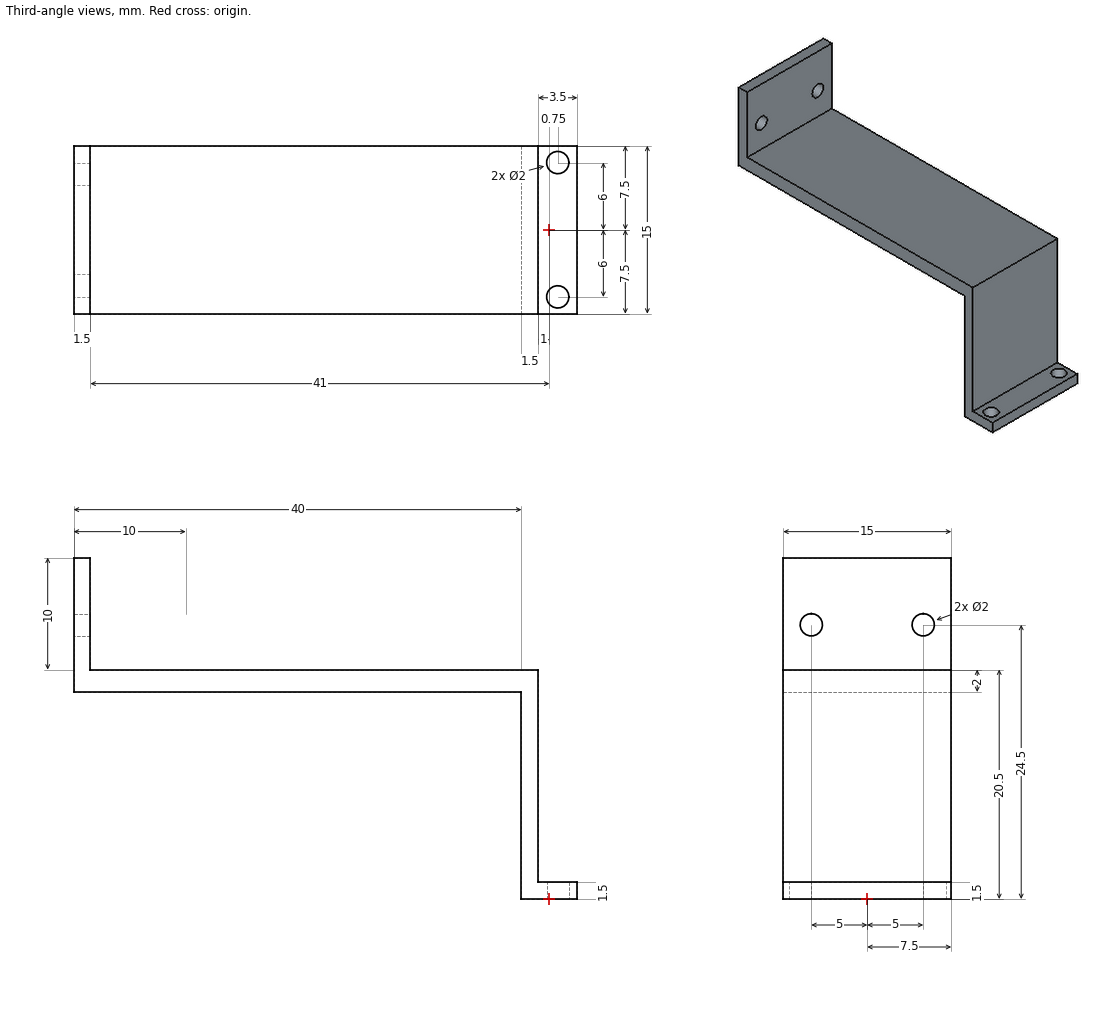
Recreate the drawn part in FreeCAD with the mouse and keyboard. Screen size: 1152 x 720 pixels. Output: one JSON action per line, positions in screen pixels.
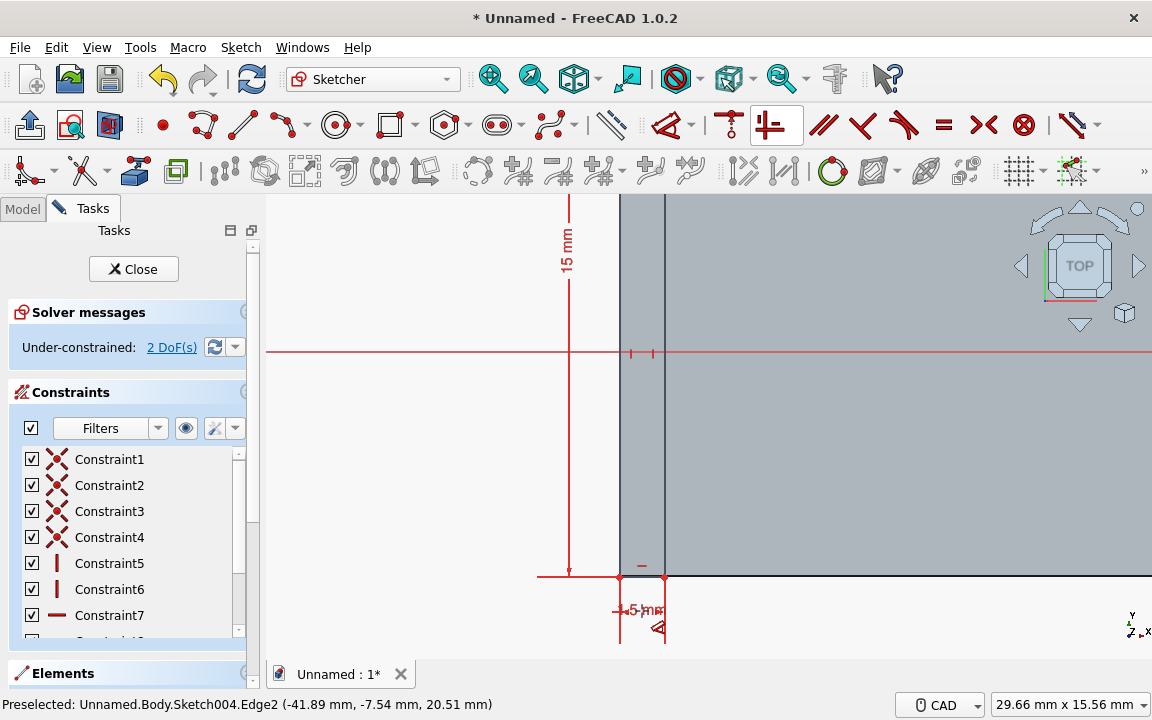
{"action": "left_click", "coordinate": [665, 577]}
{"action": "left_click", "coordinate": [826, 611]}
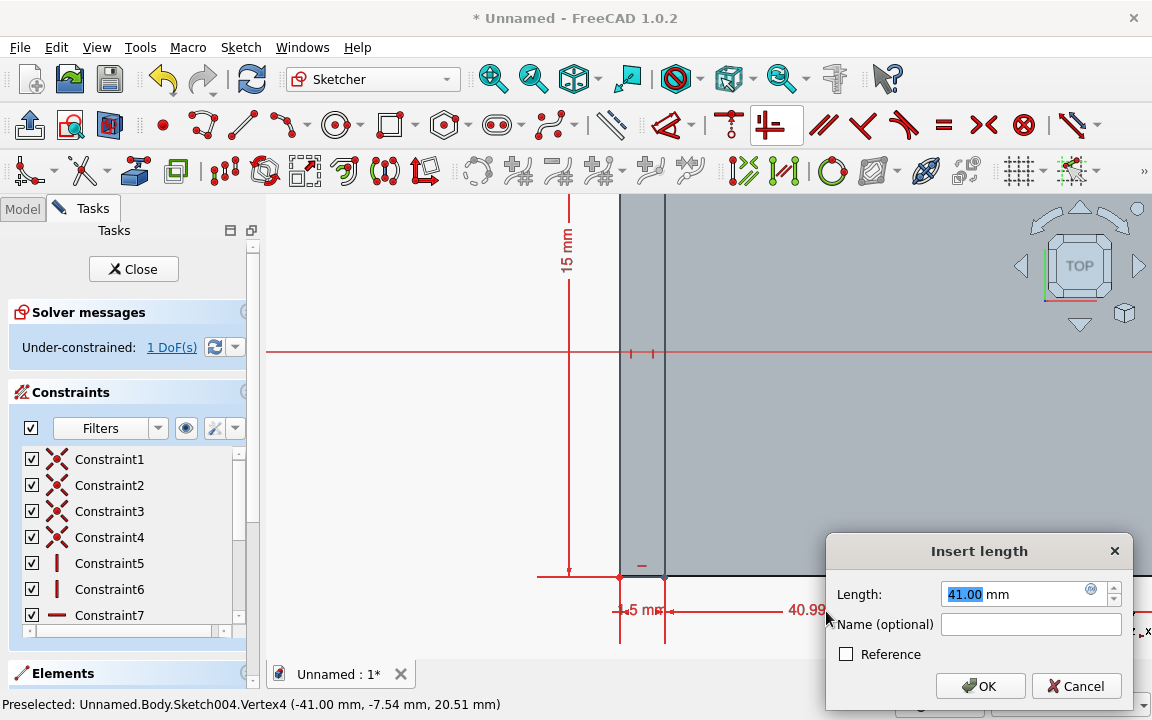
{"action": "type", "text": "41"}
{"action": "key", "text": "Return"}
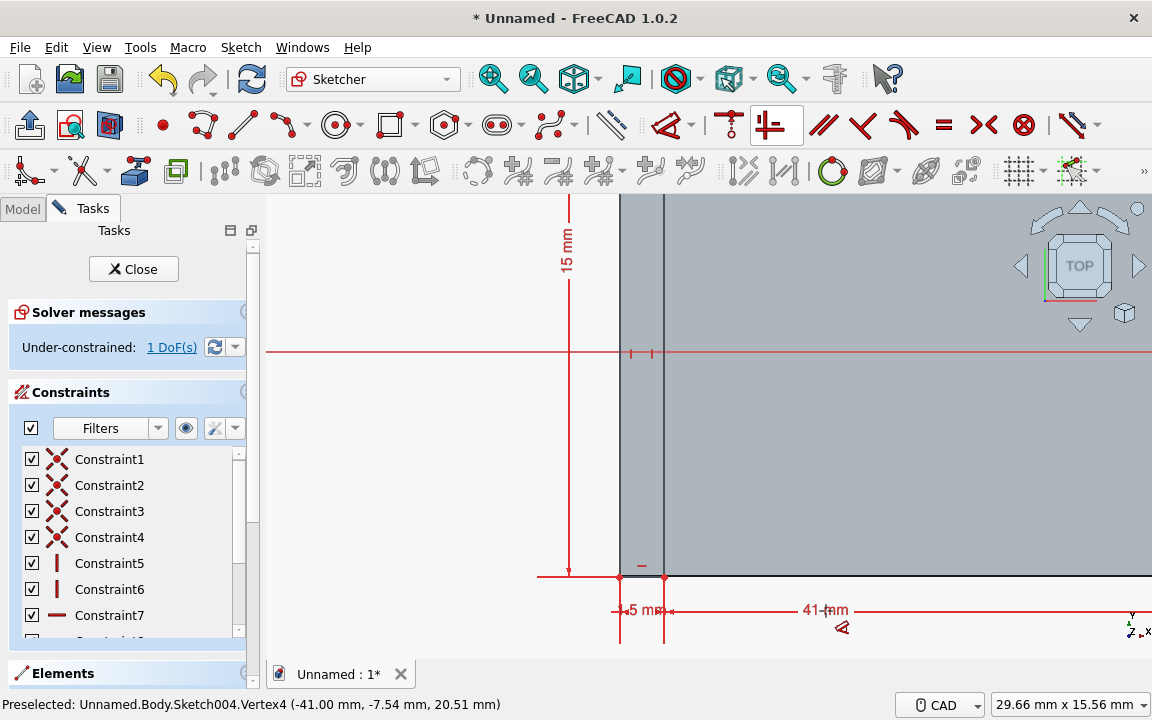
{"action": "scroll", "coordinate": [637, 578], "scroll_direction": "down", "scroll_amount": 2}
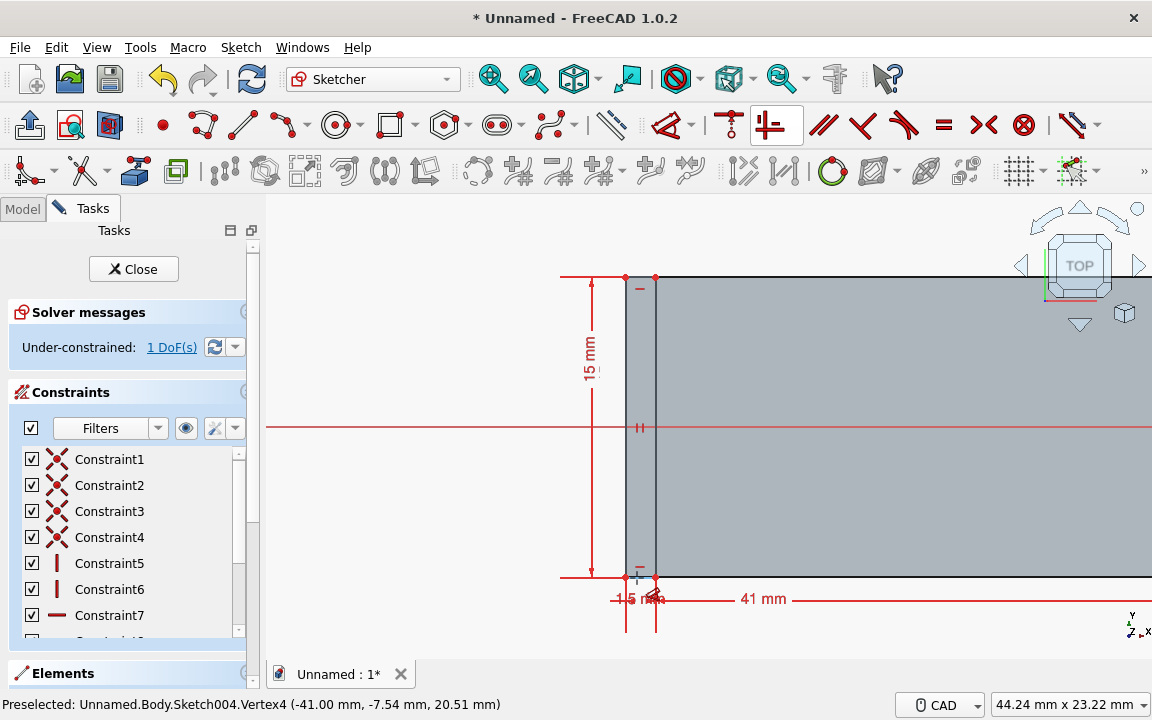
{"action": "left_click", "coordinate": [626, 277]}
{"action": "left_click", "coordinate": [592, 318]}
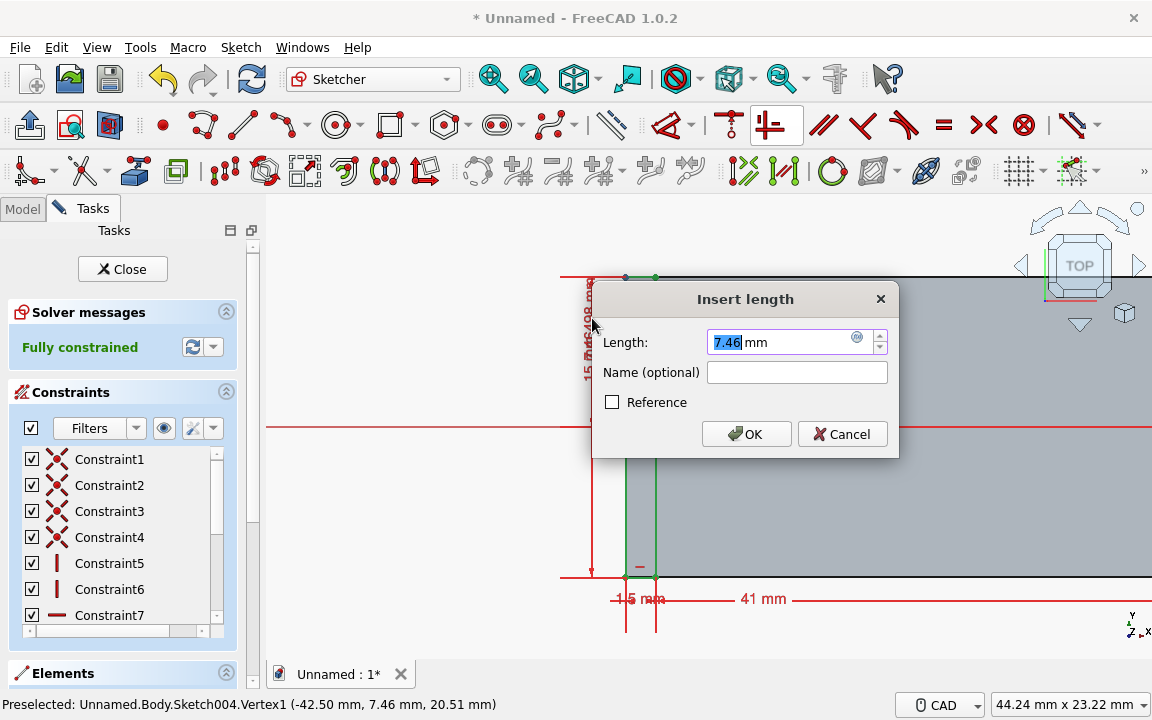
{"action": "type", "text": "7.5"}
{"action": "key", "text": "Return"}
{"action": "key", "text": "Escape"}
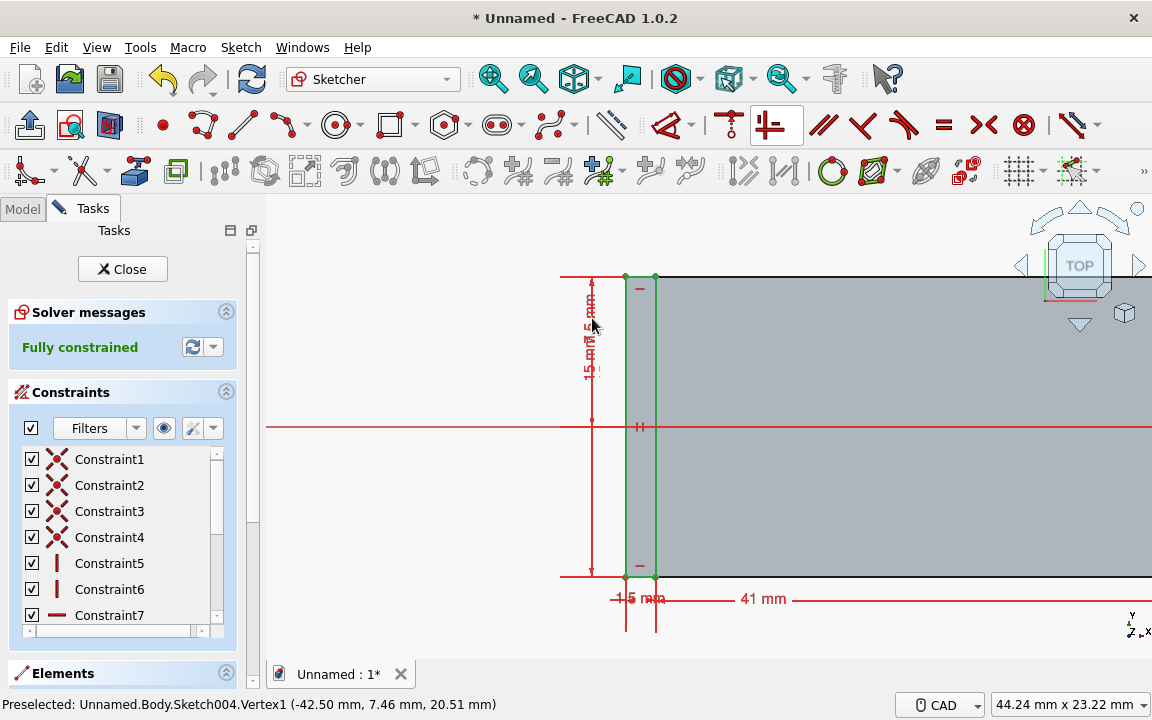
{"action": "left_click", "coordinate": [123, 269]}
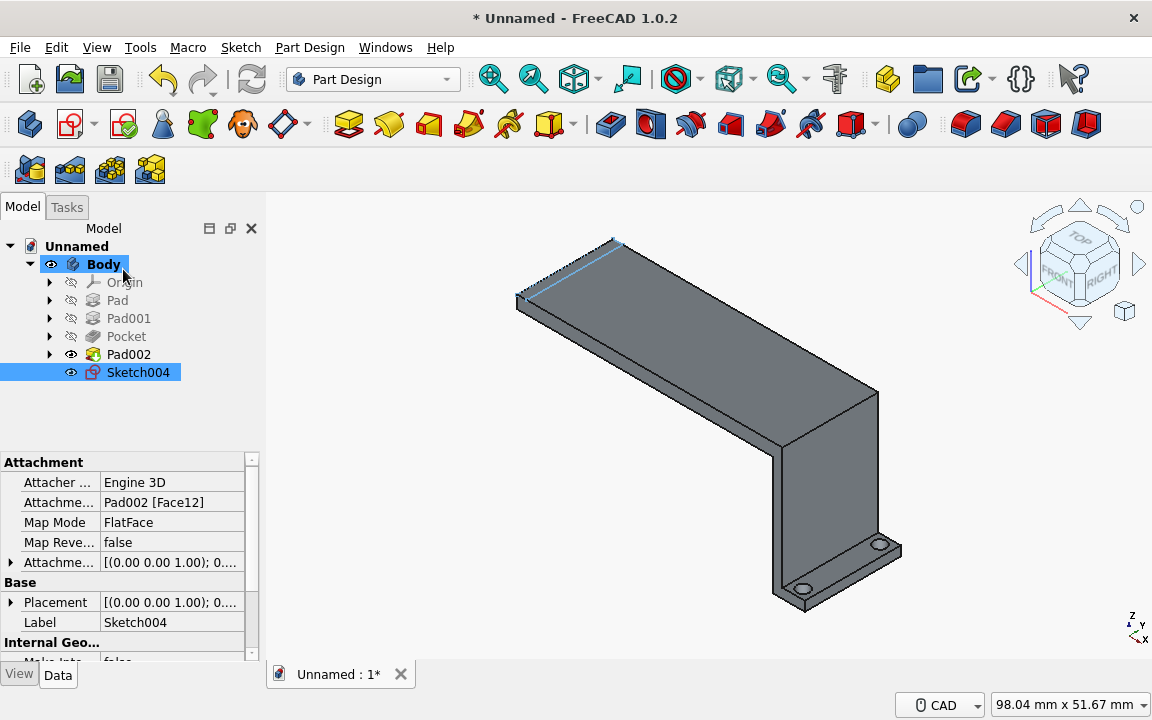
{"action": "left_click", "coordinate": [350, 124]}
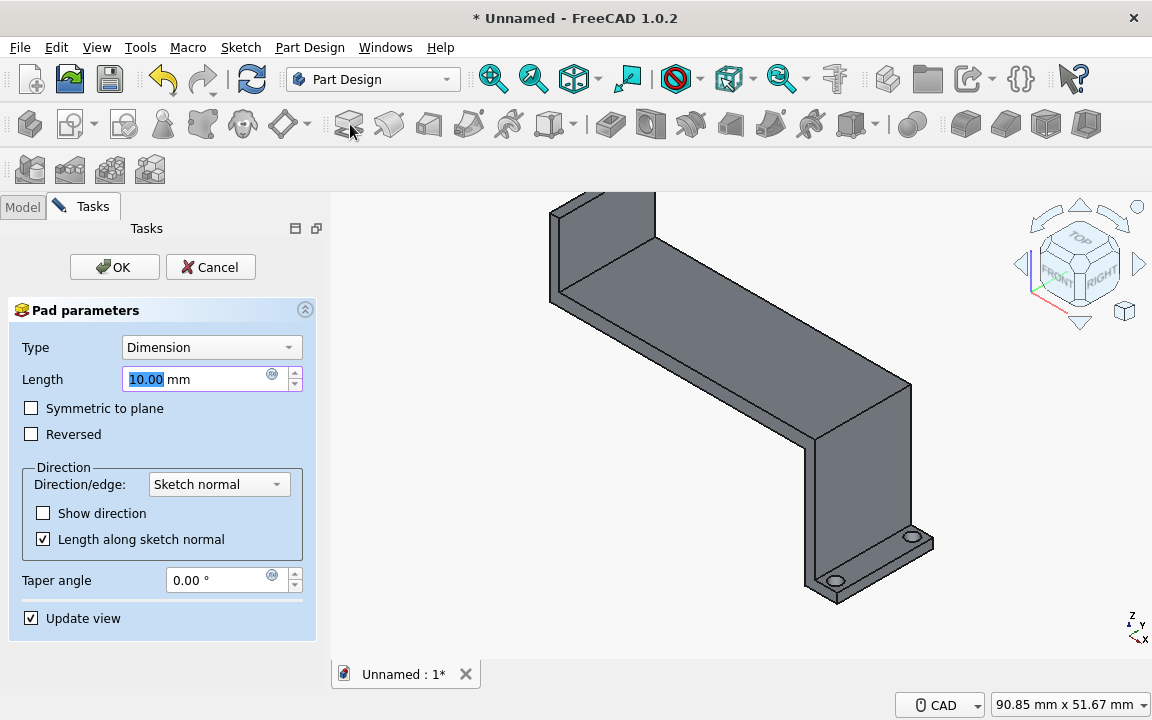
{"action": "type", "text": "10"}
{"action": "key", "text": "Tab"}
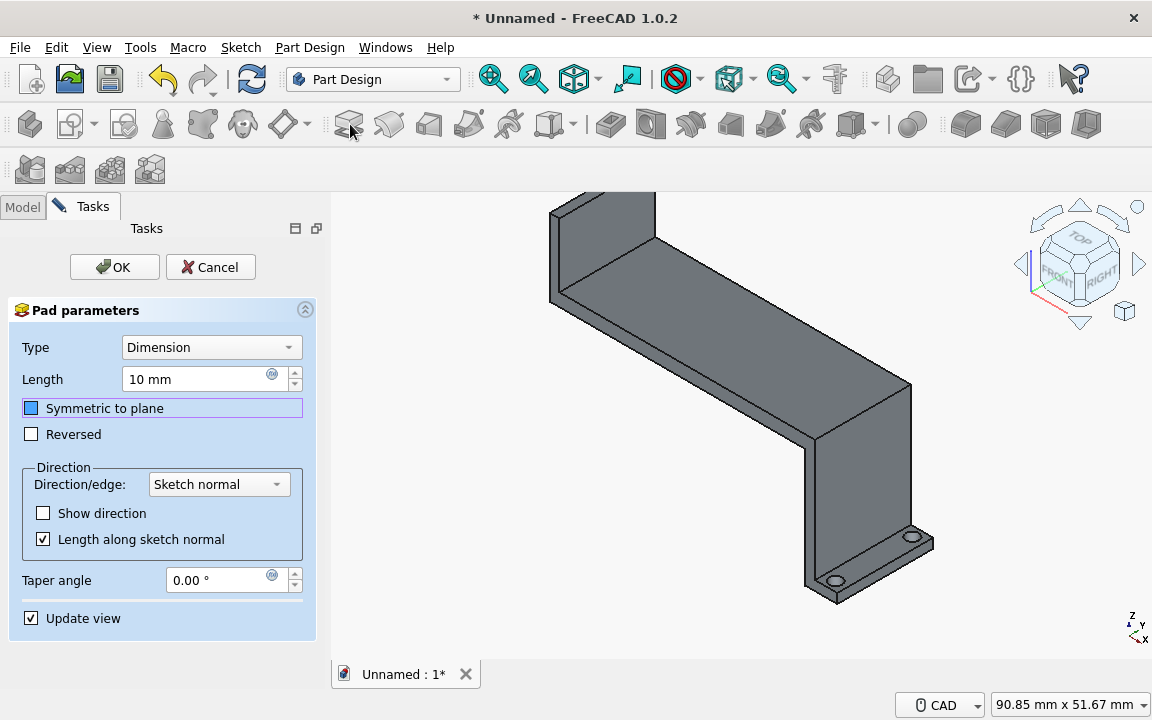
{"action": "left_click", "coordinate": [115, 267]}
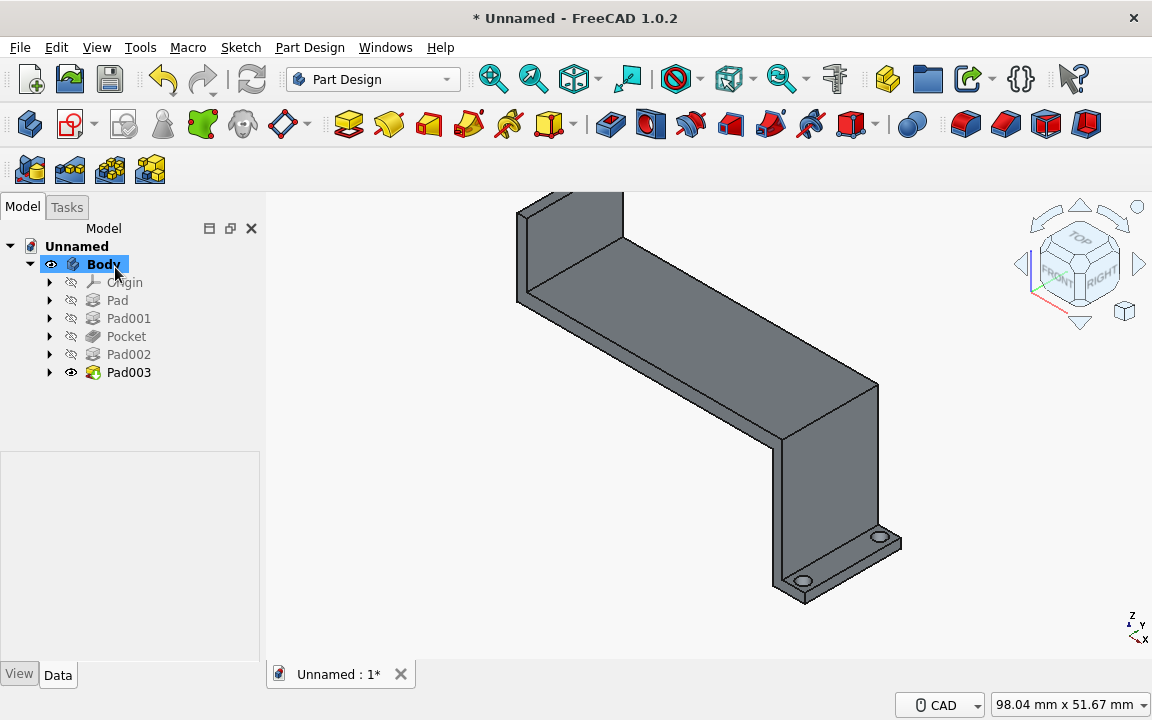
{"action": "left_click", "coordinate": [494, 80]}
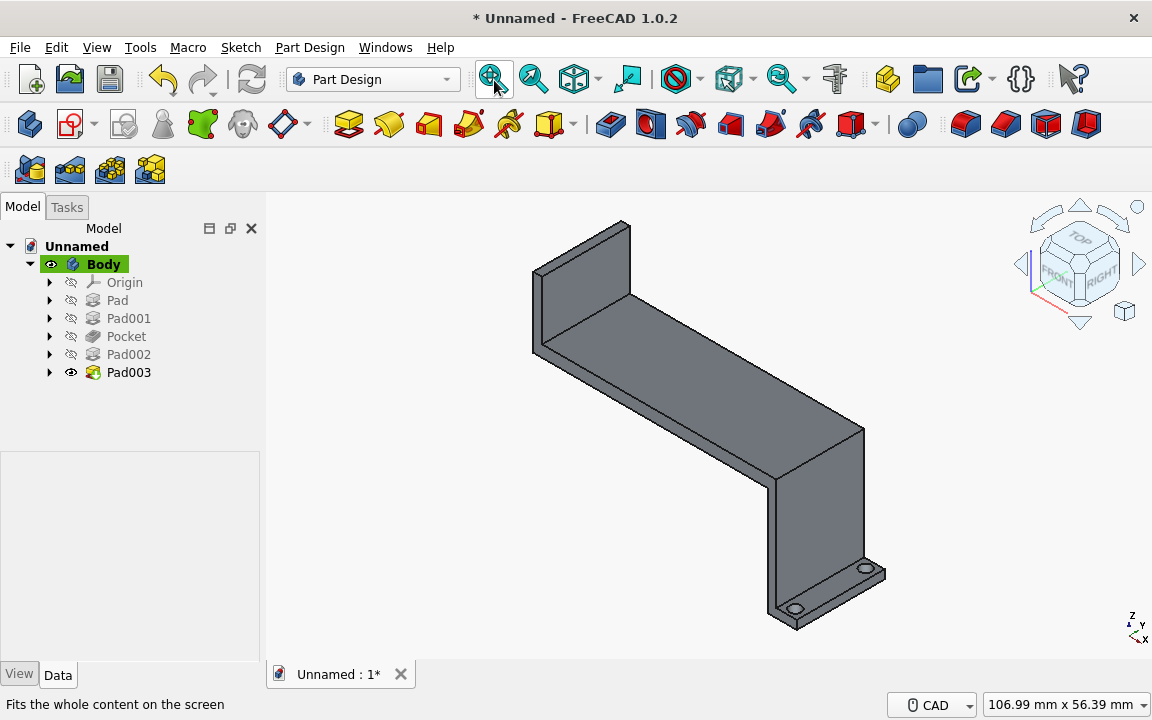
{"action": "key", "text": "6"}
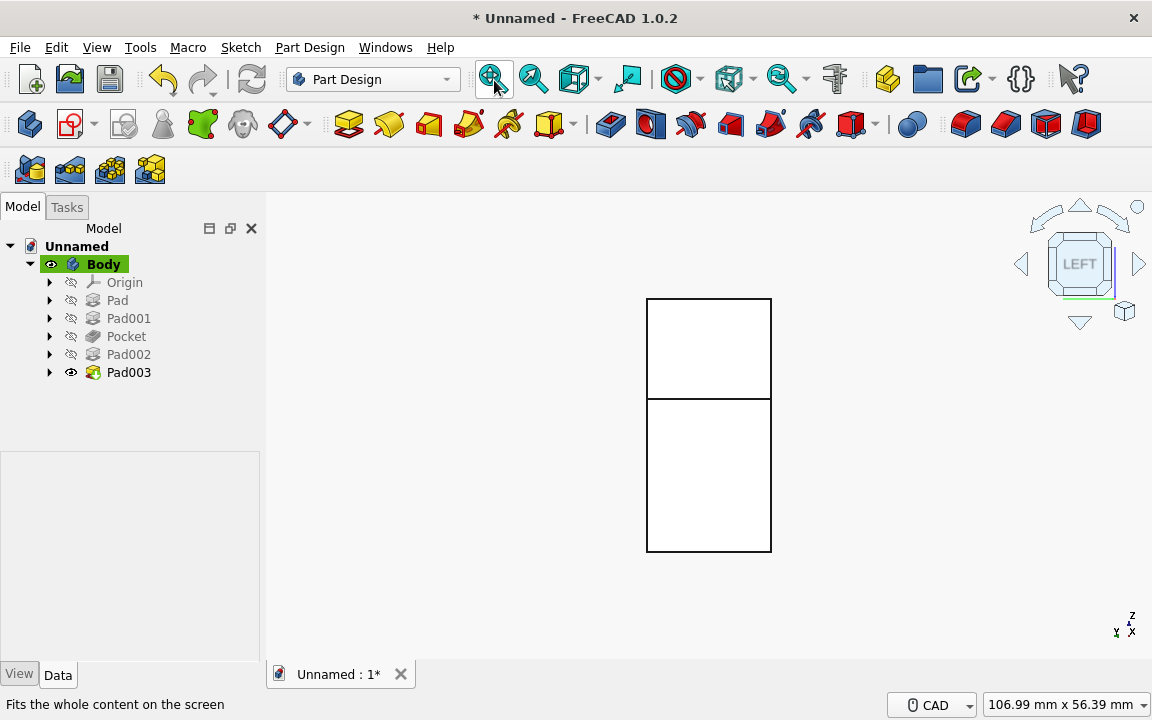
{"action": "left_click", "coordinate": [709, 348]}